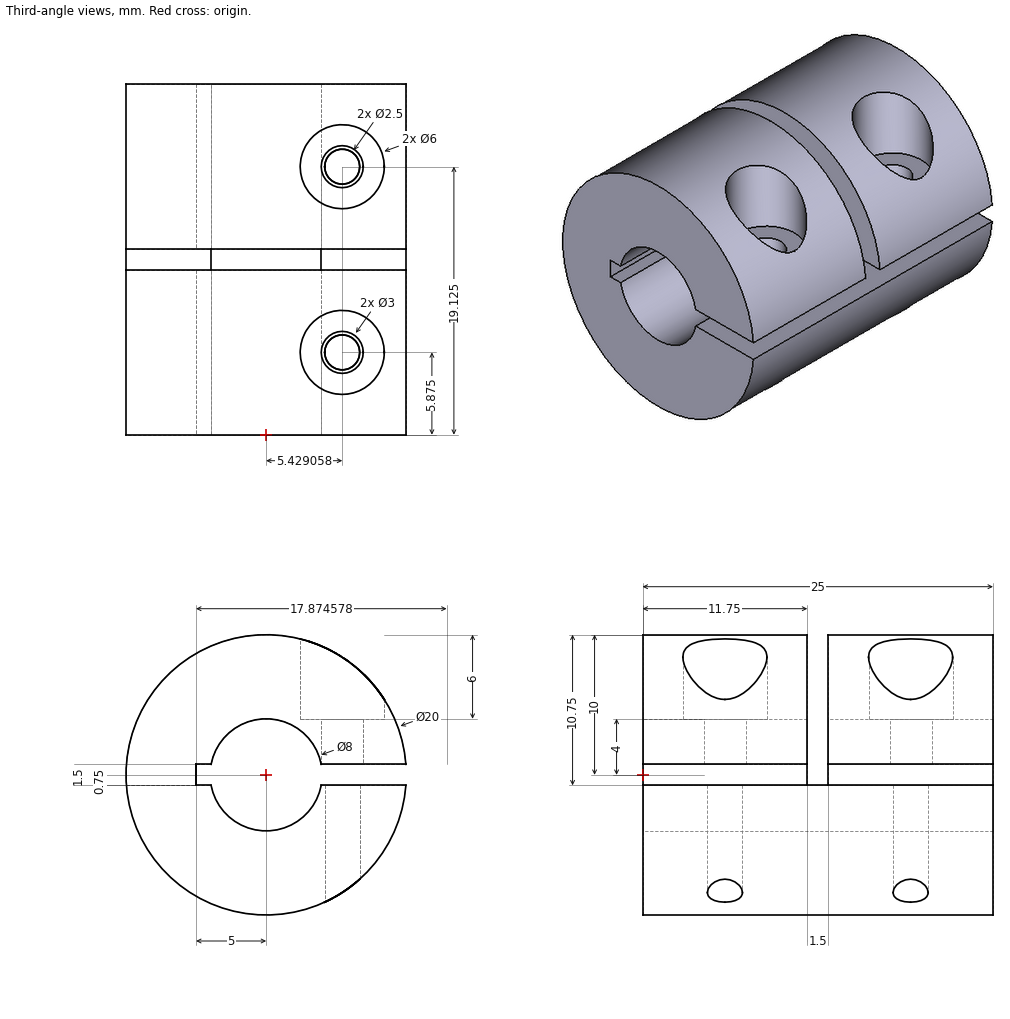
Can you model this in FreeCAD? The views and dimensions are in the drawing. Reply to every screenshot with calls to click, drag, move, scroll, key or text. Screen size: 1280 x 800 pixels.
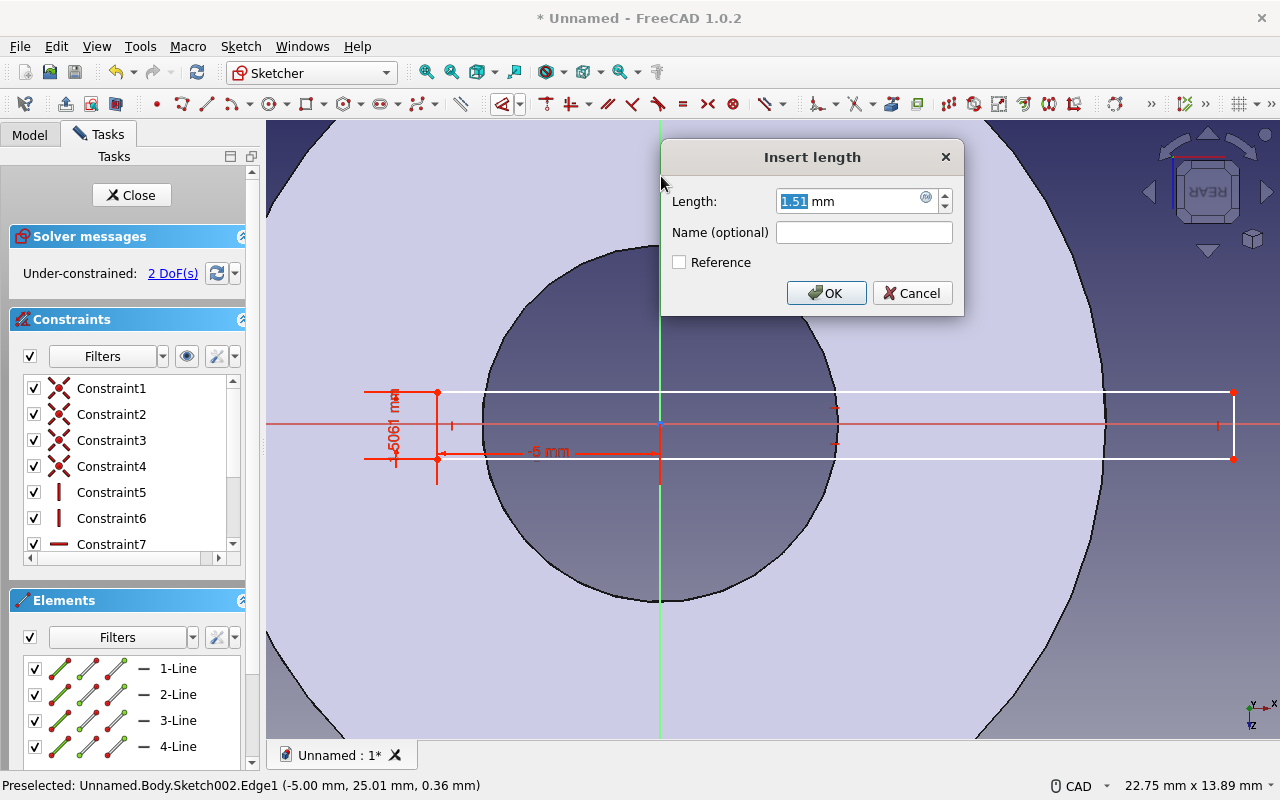
text(1.5)
key(Return)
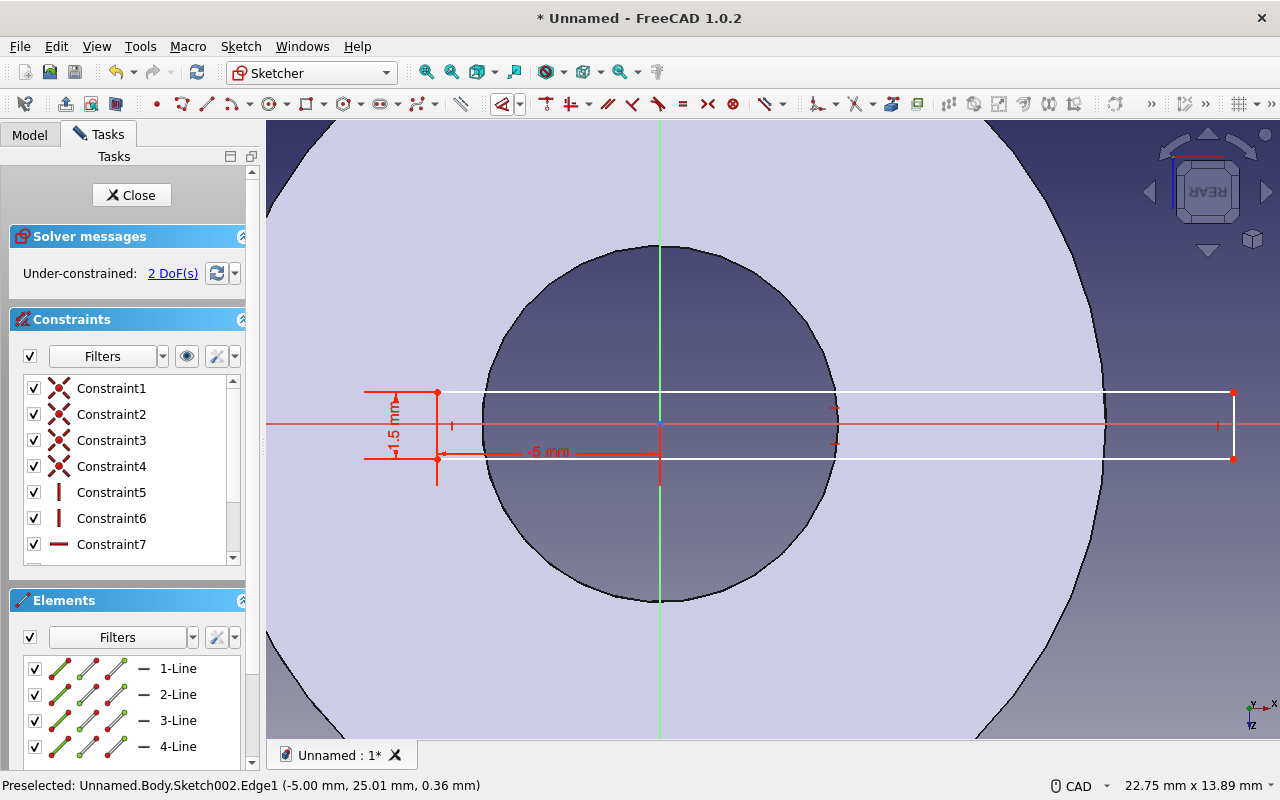
click(437, 392)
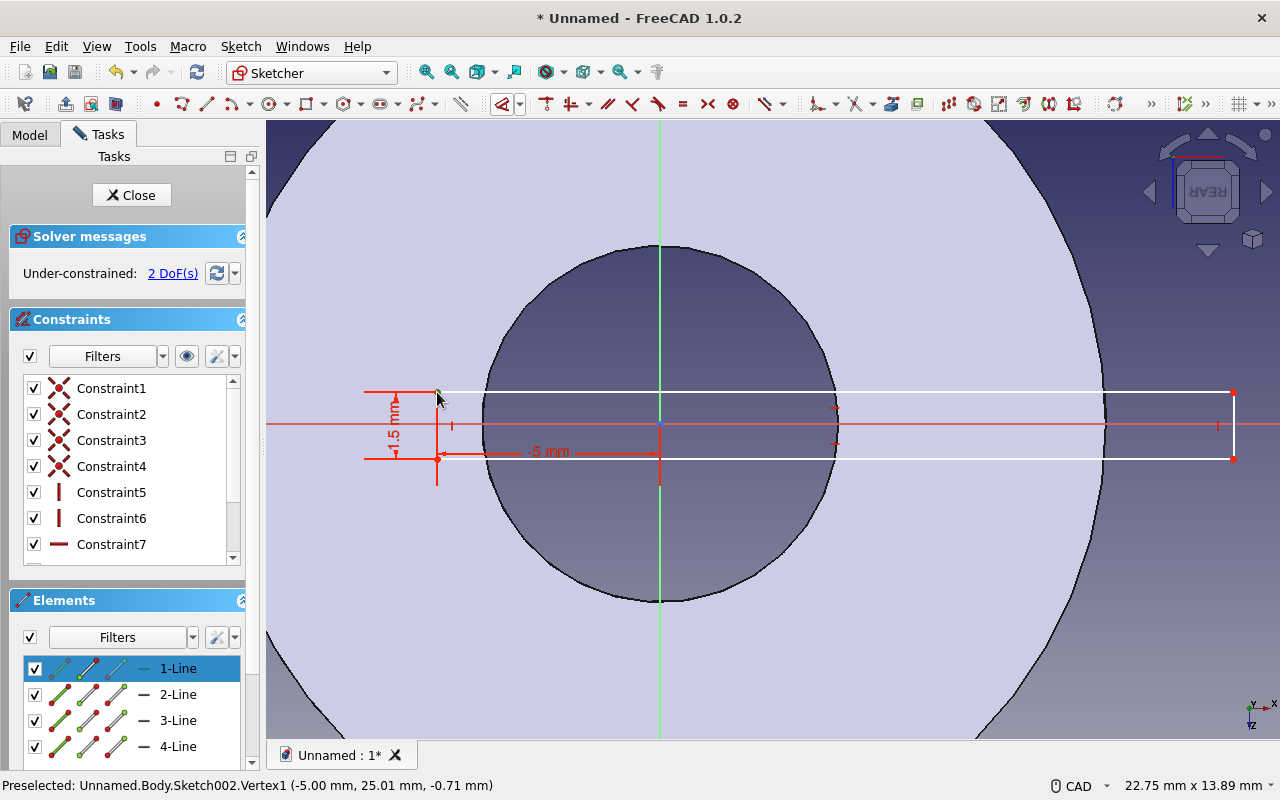
click(520, 104)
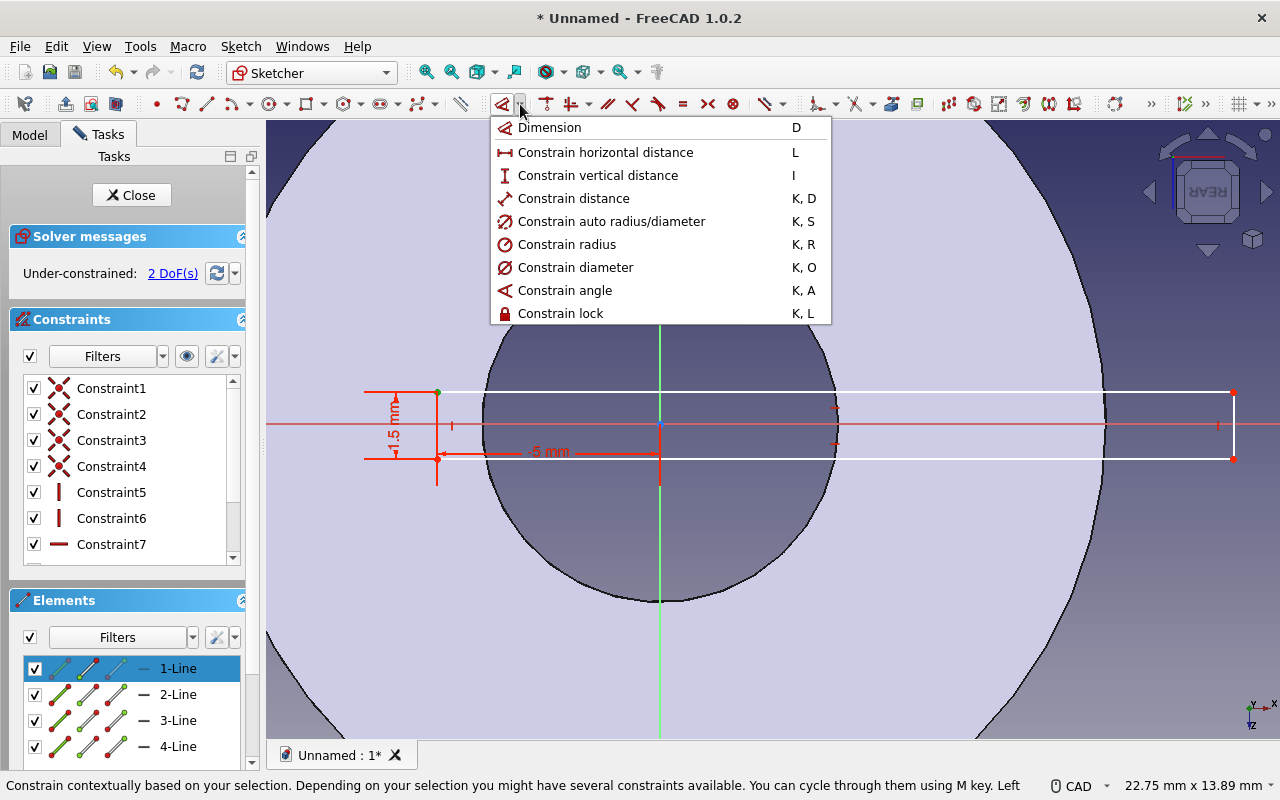
click(661, 176)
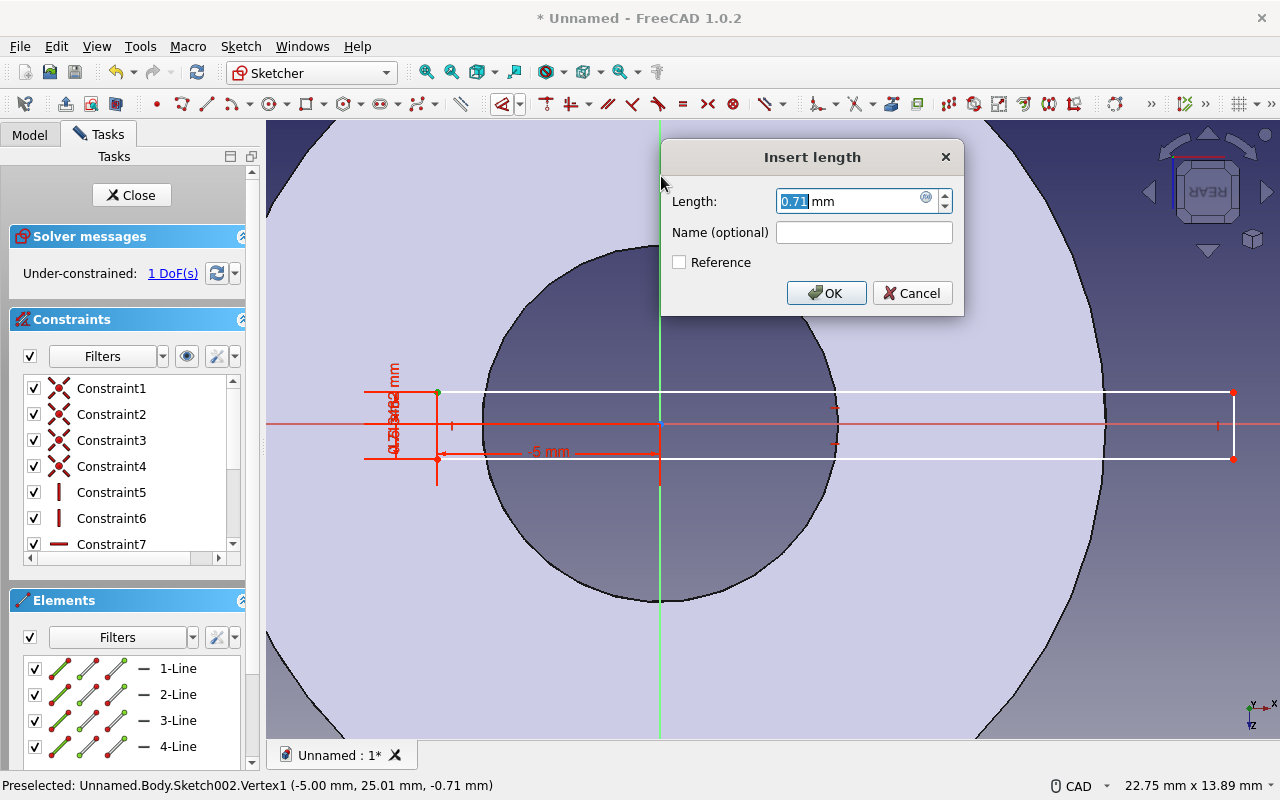
text(0.75)
key(Return)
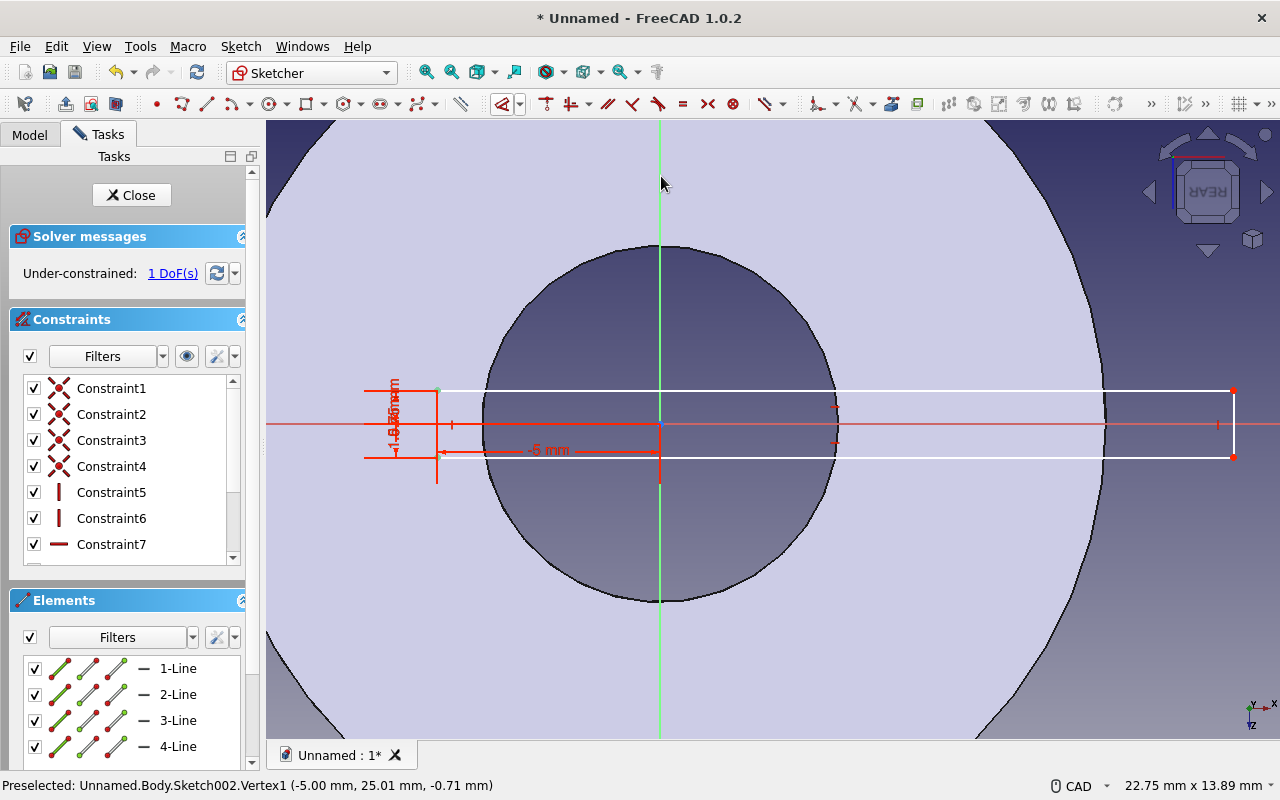
click(676, 458)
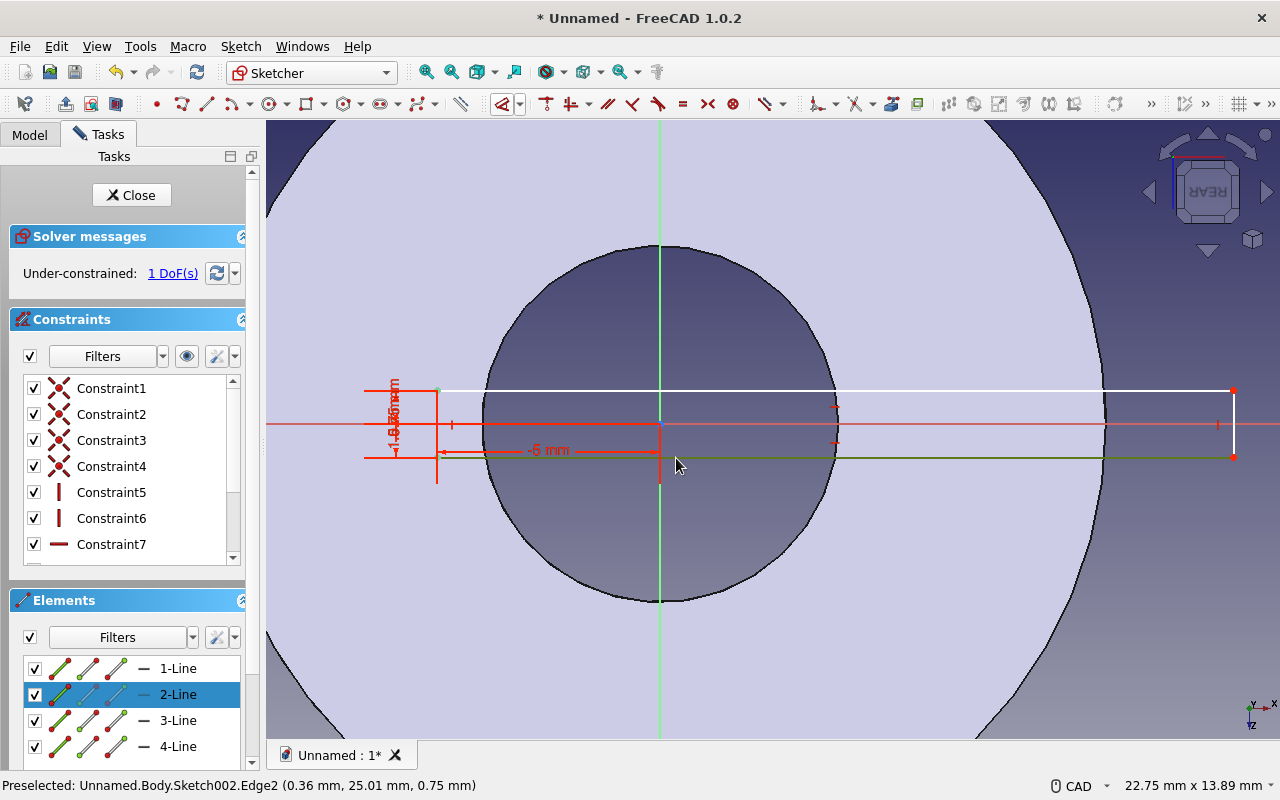
click(520, 104)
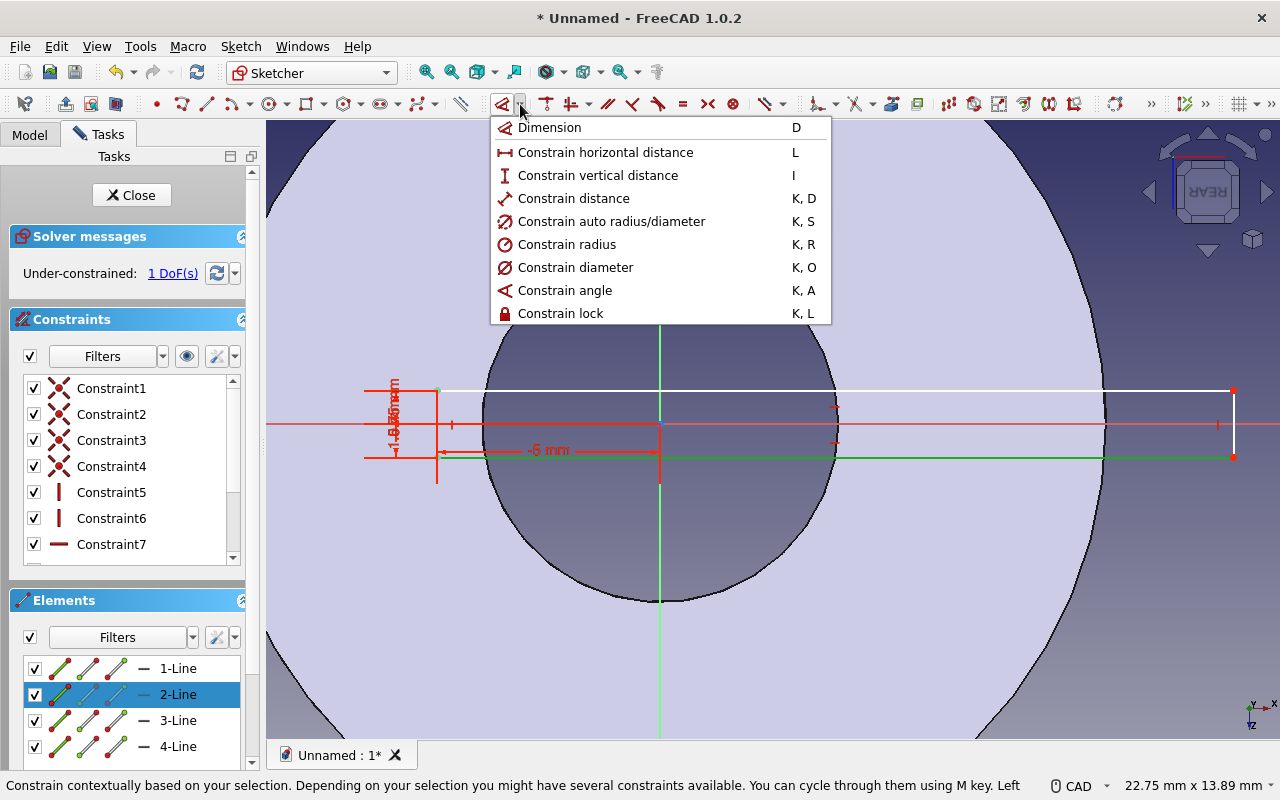
click(661, 152)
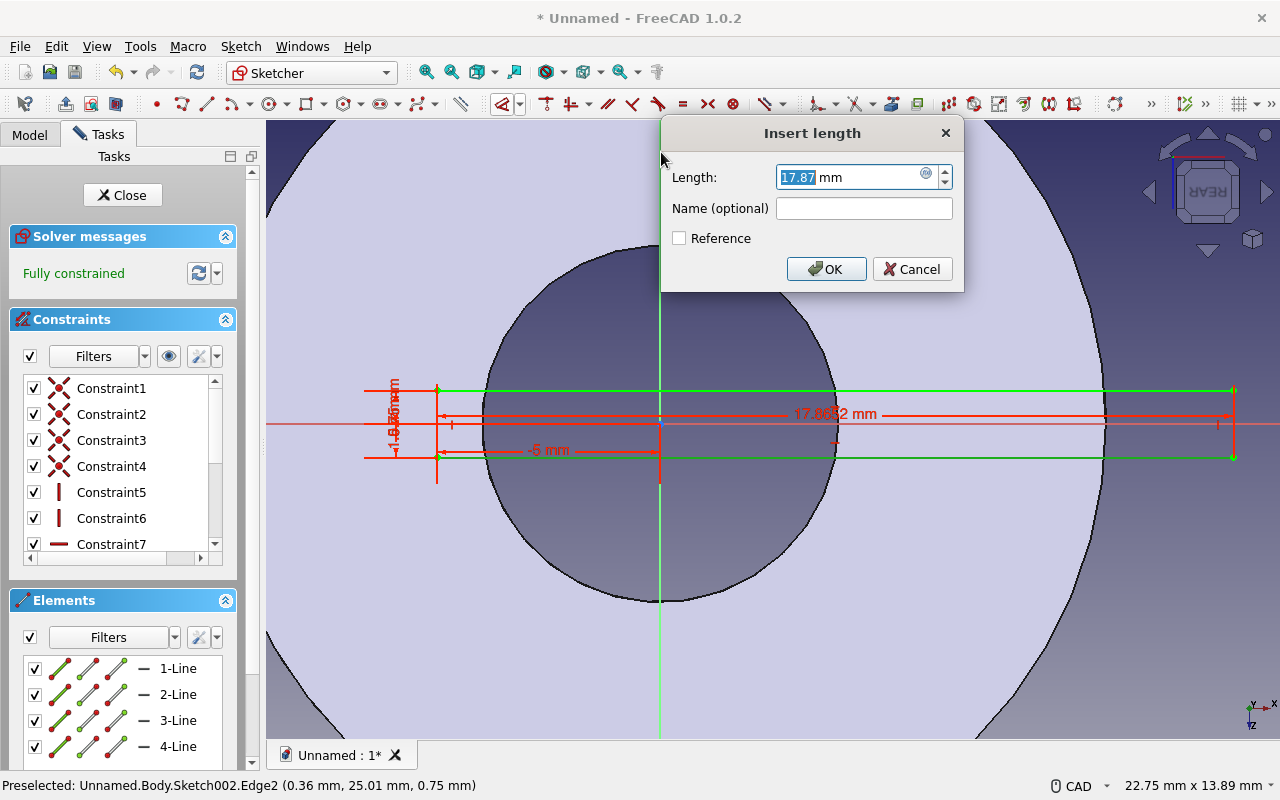
text(17.874578)
key(Return)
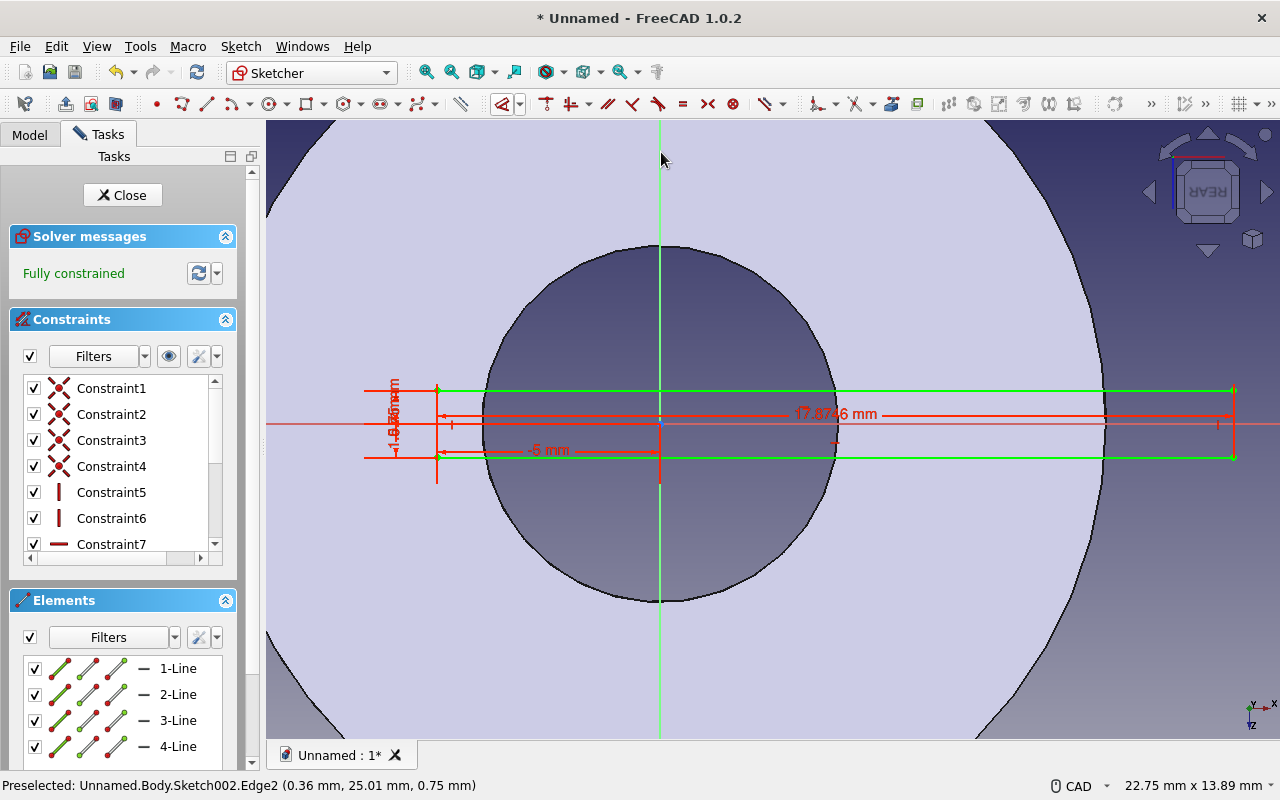
click(123, 195)